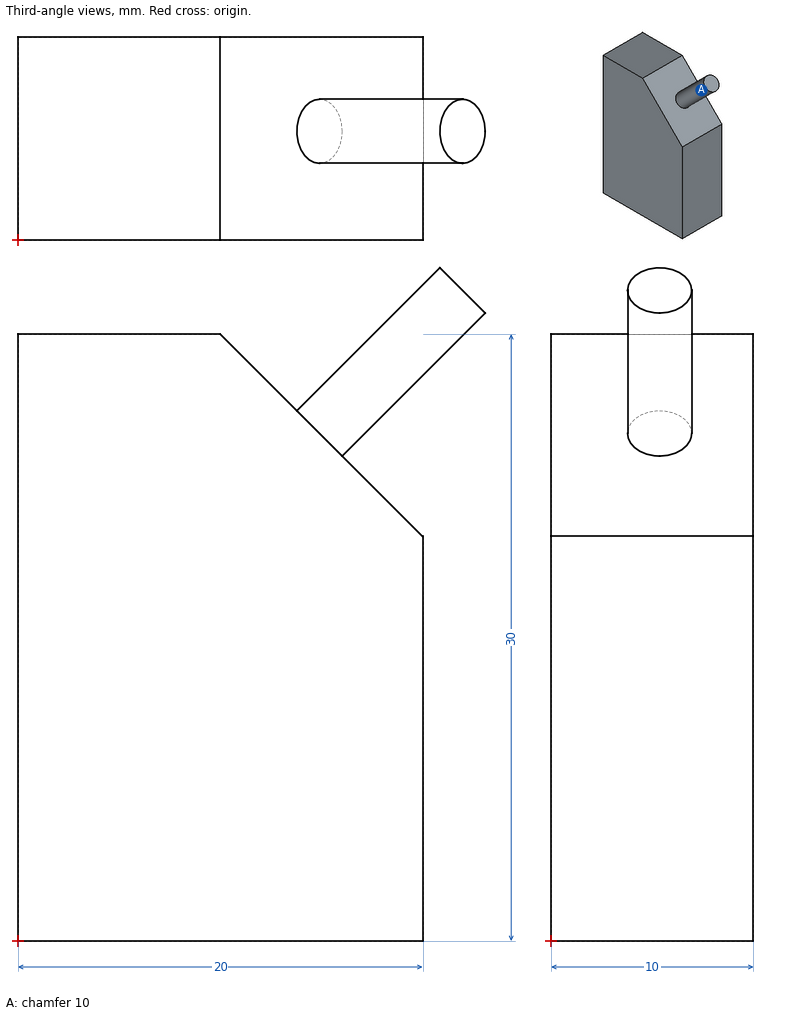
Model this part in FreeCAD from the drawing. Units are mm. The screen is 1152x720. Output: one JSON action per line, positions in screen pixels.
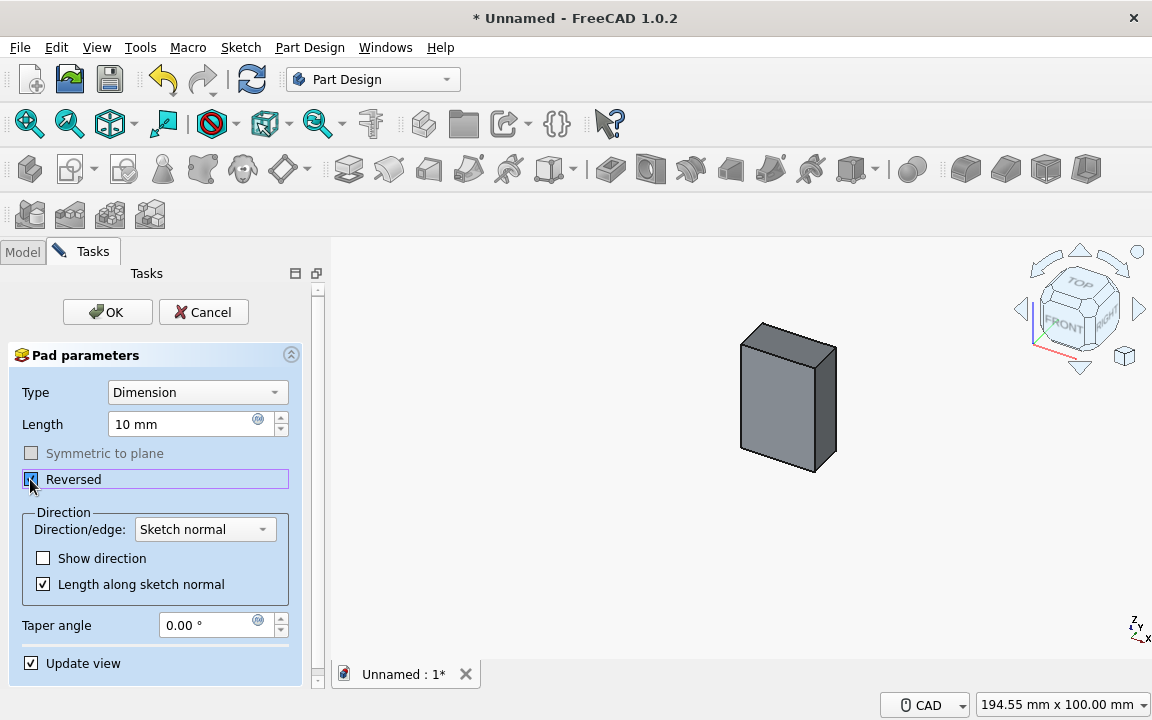
{"action": "left_click", "coordinate": [108, 312]}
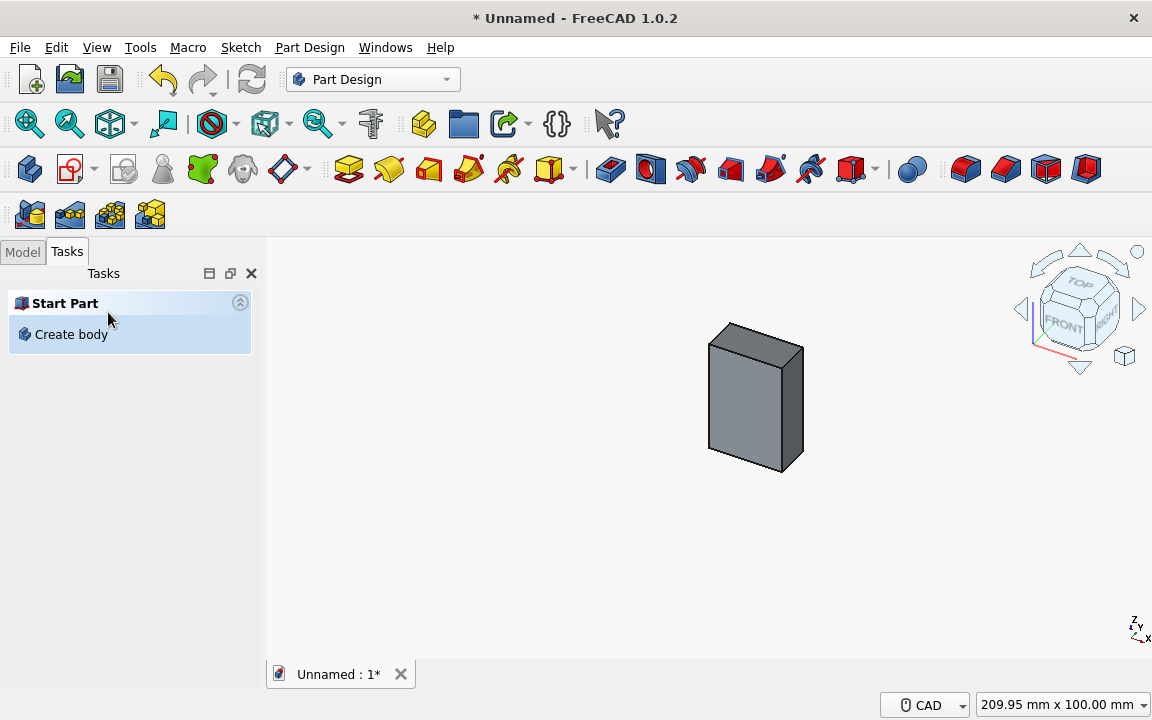
{"action": "left_click", "coordinate": [30, 124]}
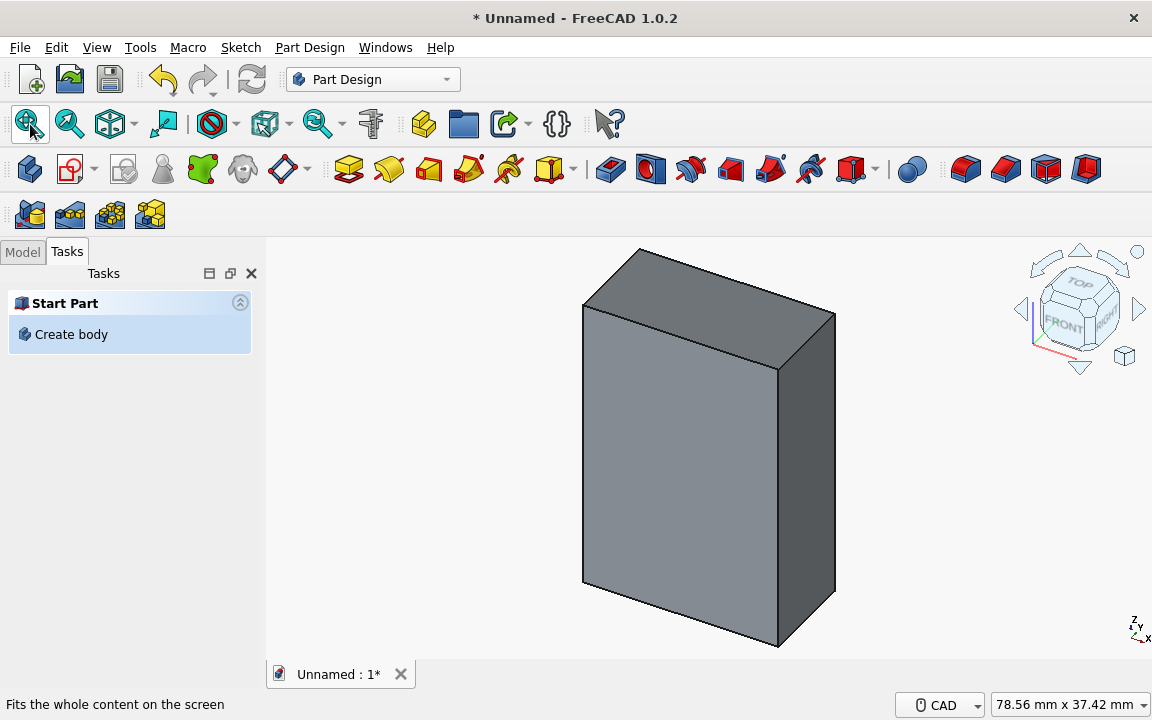
{"action": "left_click", "coordinate": [807, 341]}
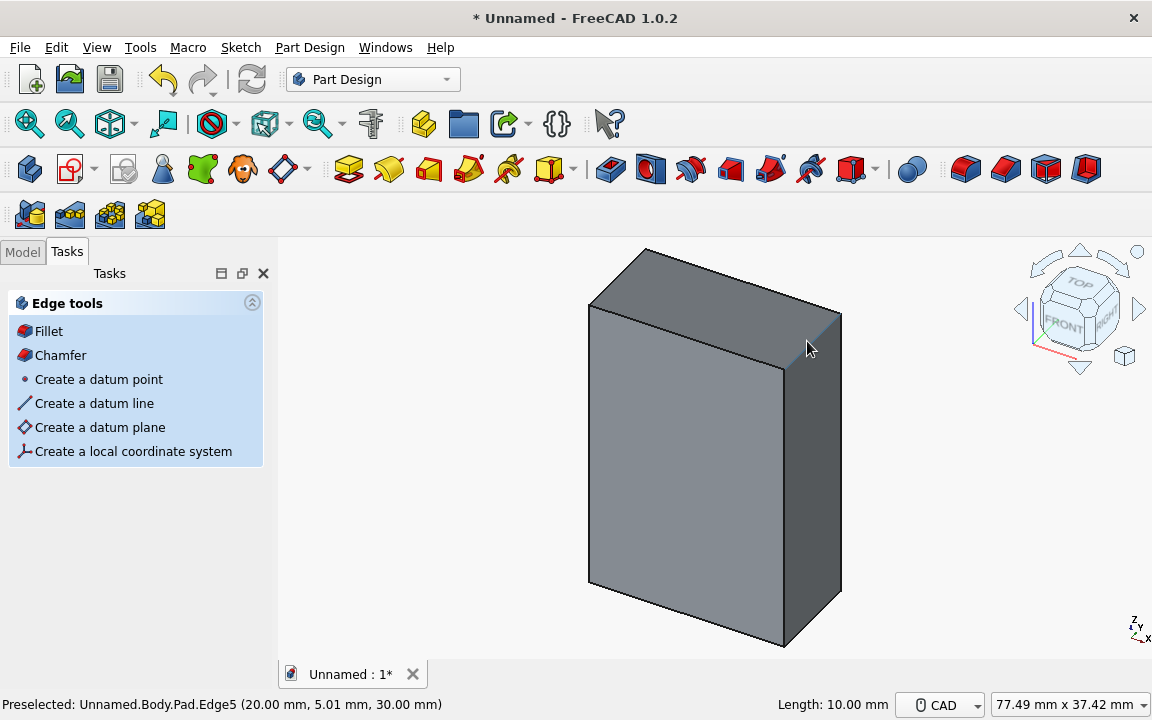
{"action": "left_click", "coordinate": [1006, 170]}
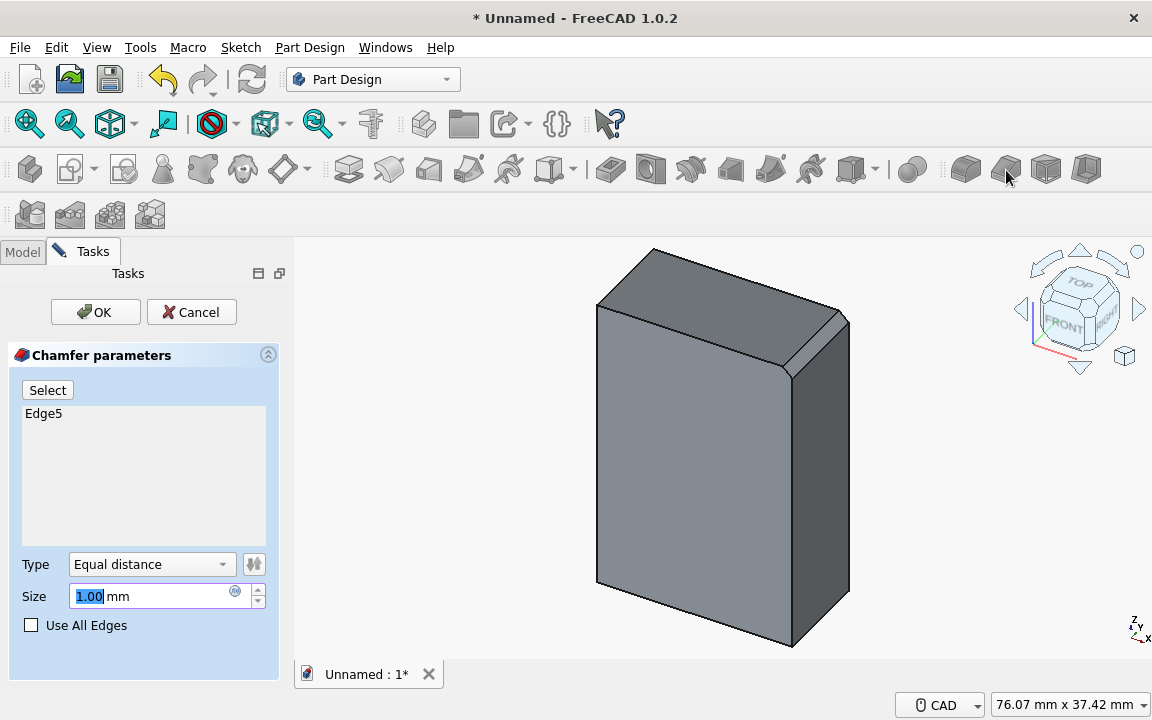
{"action": "type", "text": "10"}
{"action": "key", "text": "Tab"}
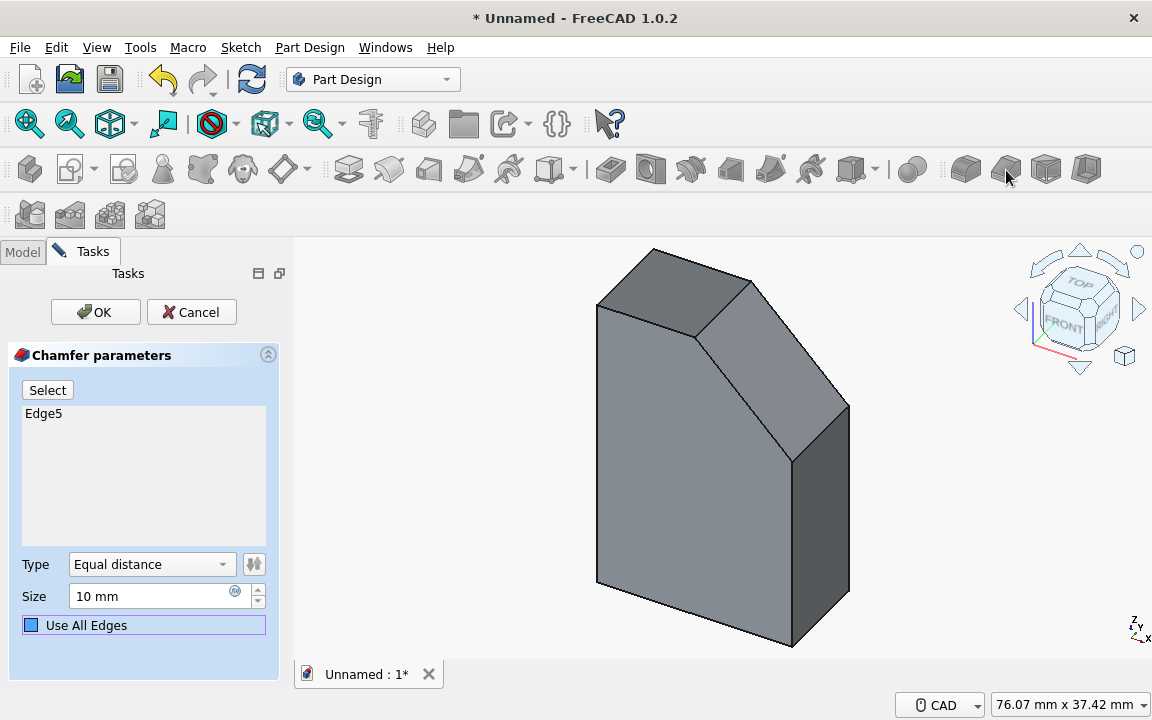
{"action": "left_click", "coordinate": [96, 312]}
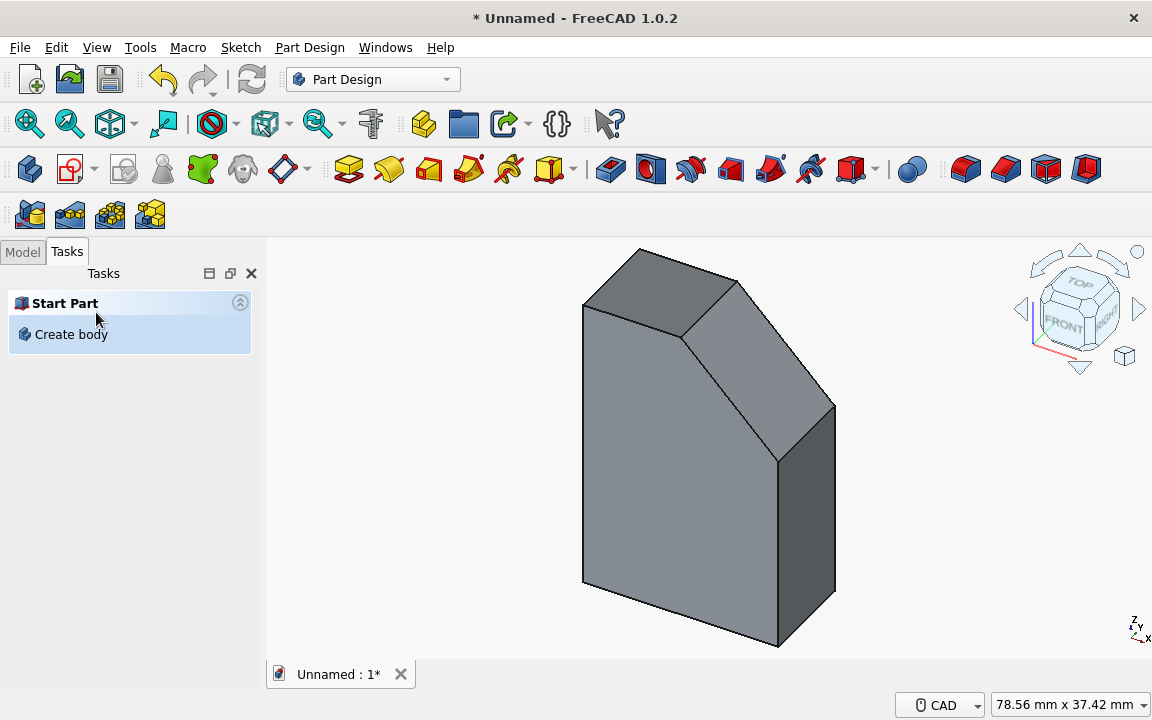
{"action": "left_click", "coordinate": [744, 353]}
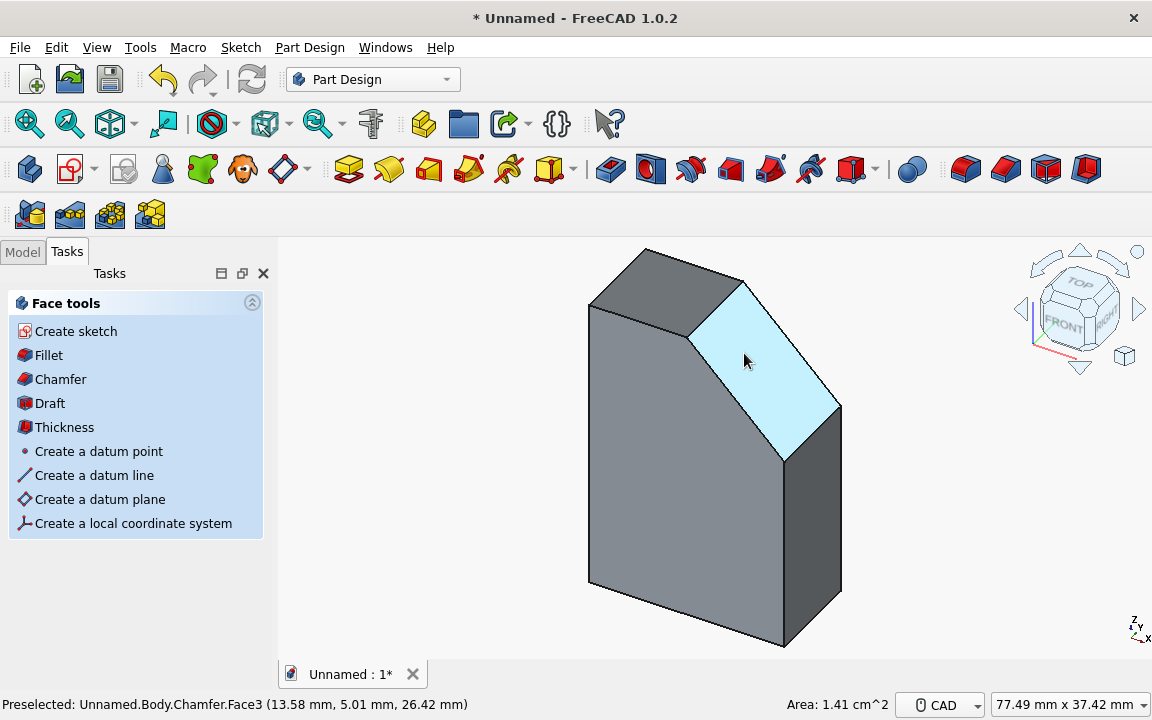
{"action": "left_click", "coordinate": [70, 170]}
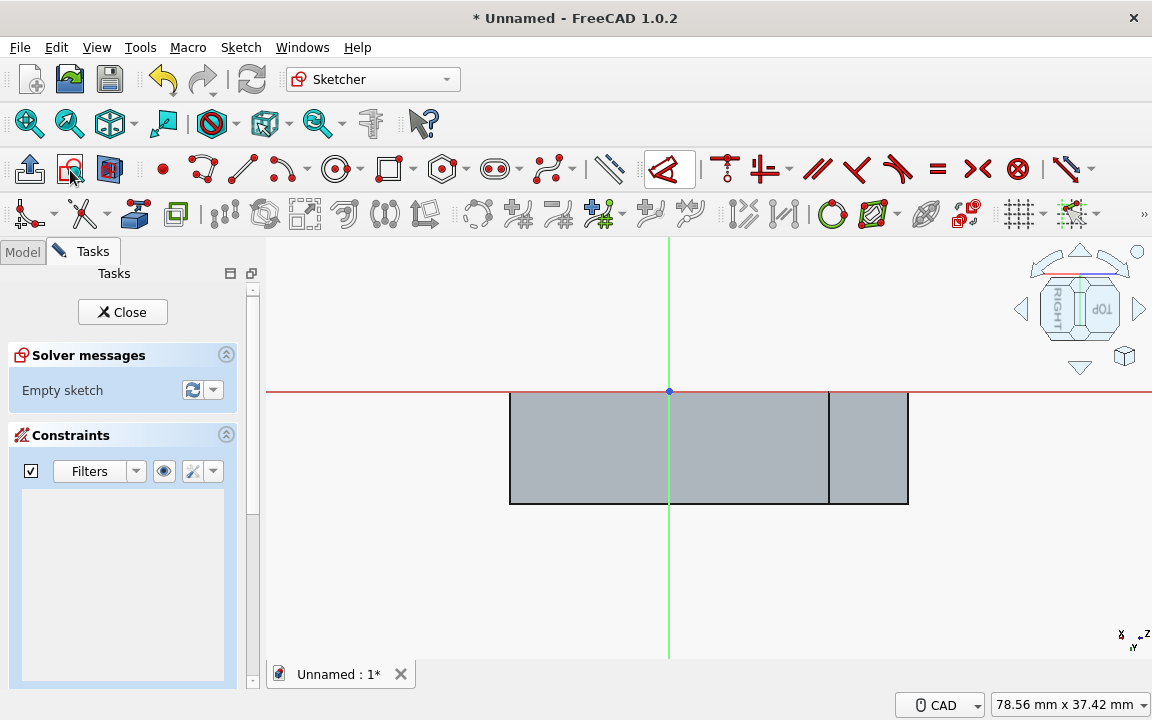
{"action": "key", "text": "q s"}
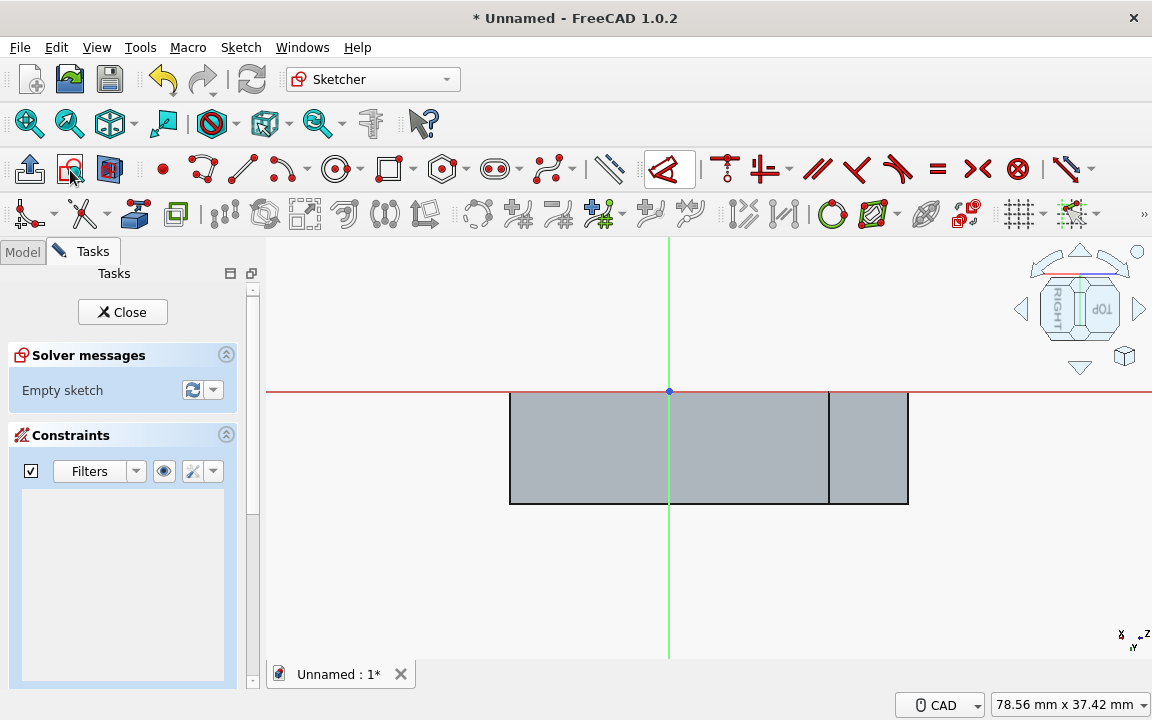
{"action": "scroll", "coordinate": [768, 453], "scroll_direction": "up", "scroll_amount": 10}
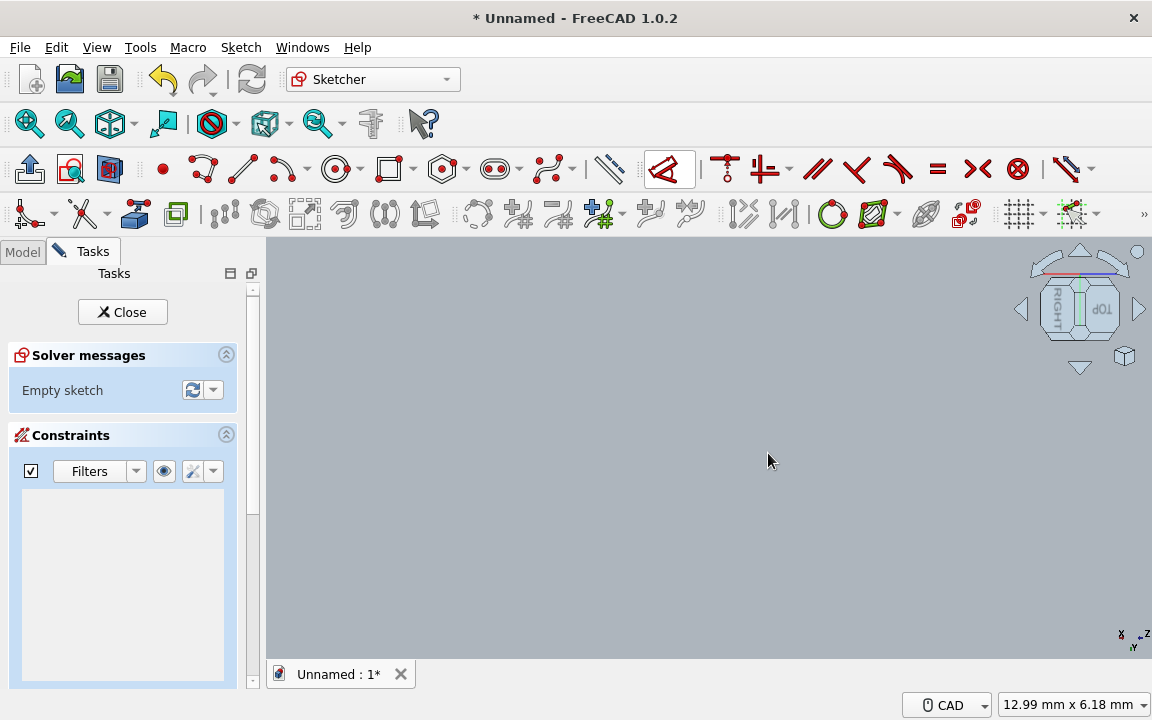
{"action": "key", "text": "g c"}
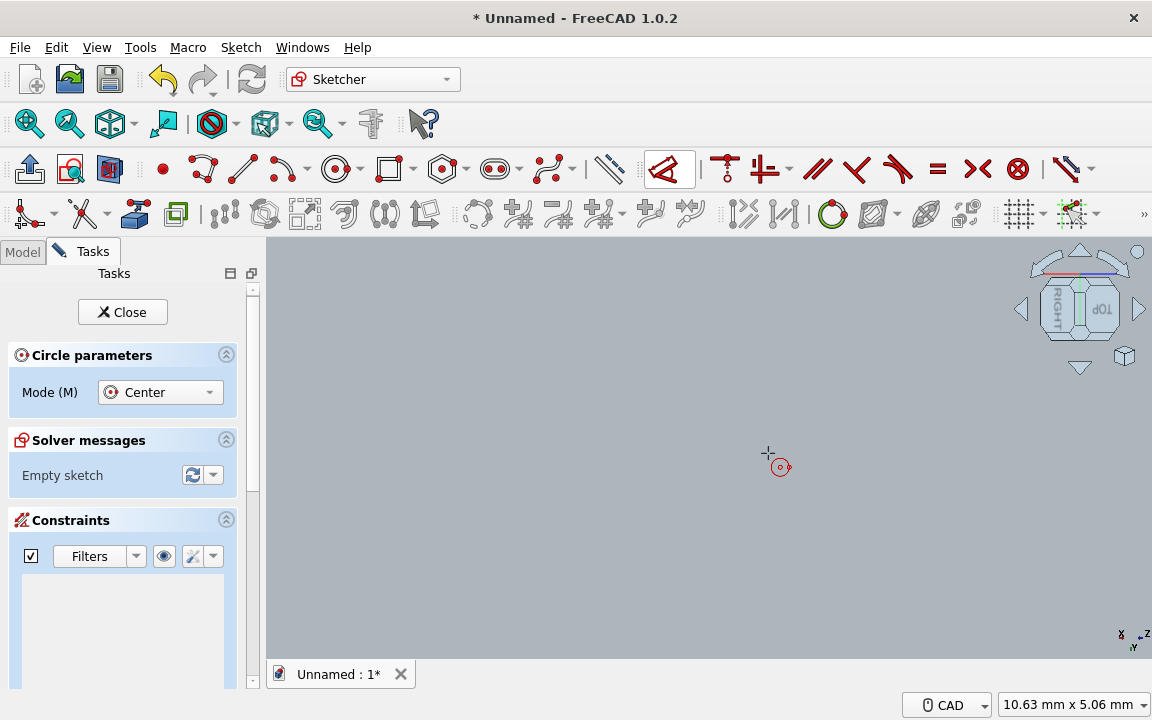
{"action": "left_click", "coordinate": [634, 443]}
{"action": "mouse_move", "coordinate": [727, 349]}